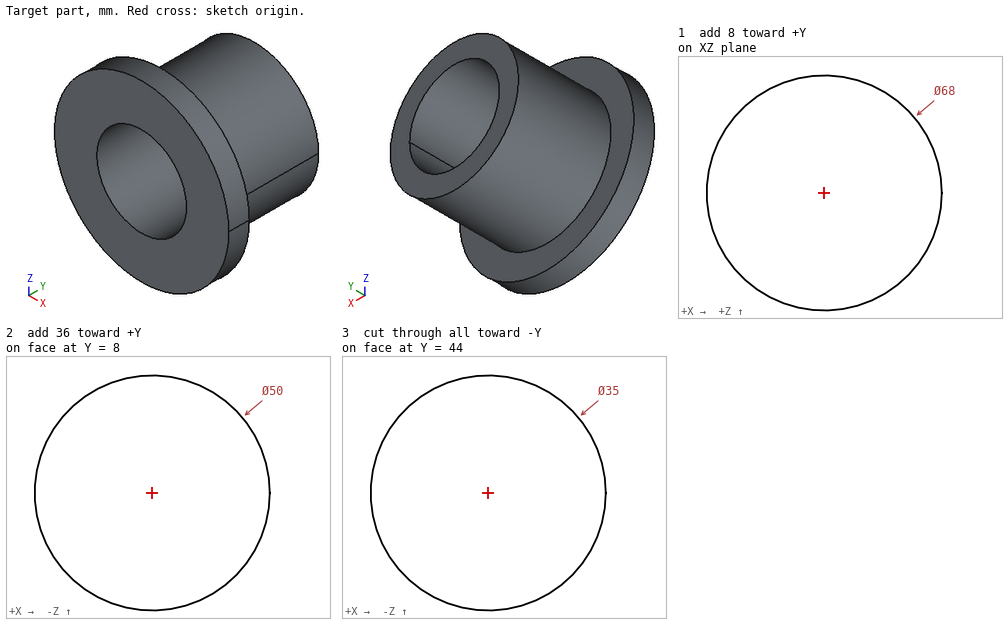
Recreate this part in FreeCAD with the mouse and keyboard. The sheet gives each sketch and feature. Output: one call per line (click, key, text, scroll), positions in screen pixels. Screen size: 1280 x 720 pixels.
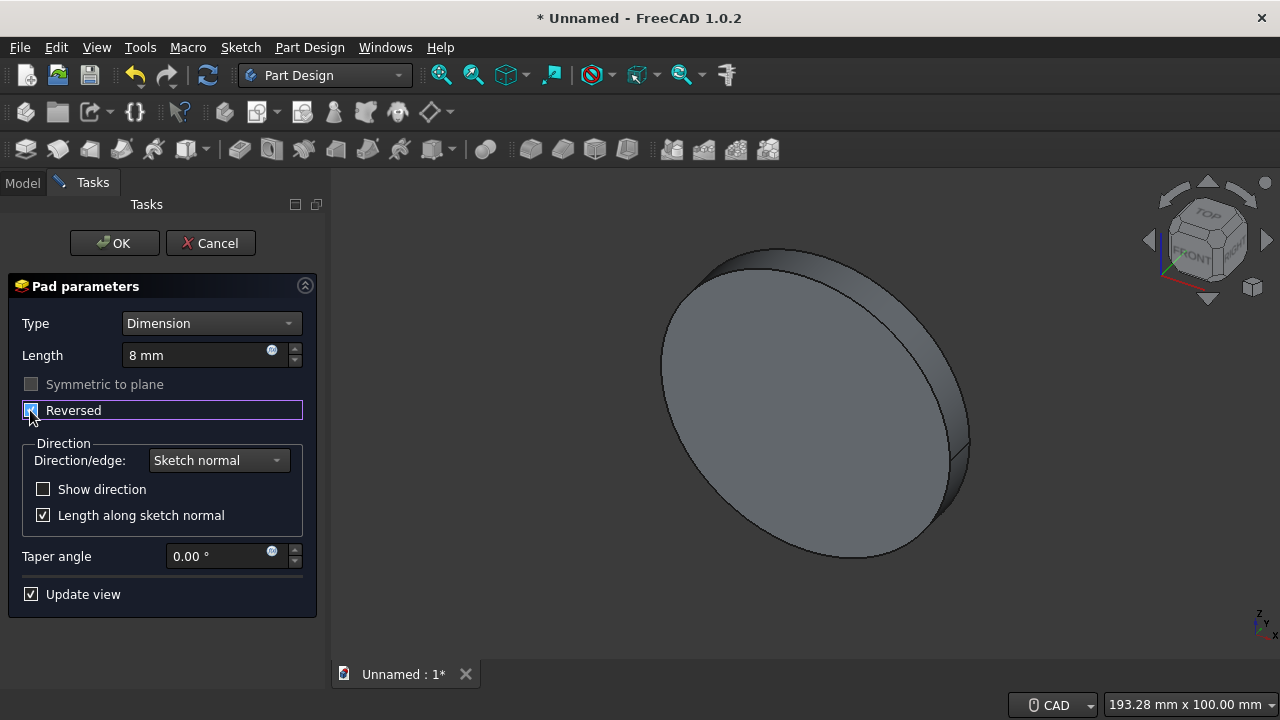
click(115, 243)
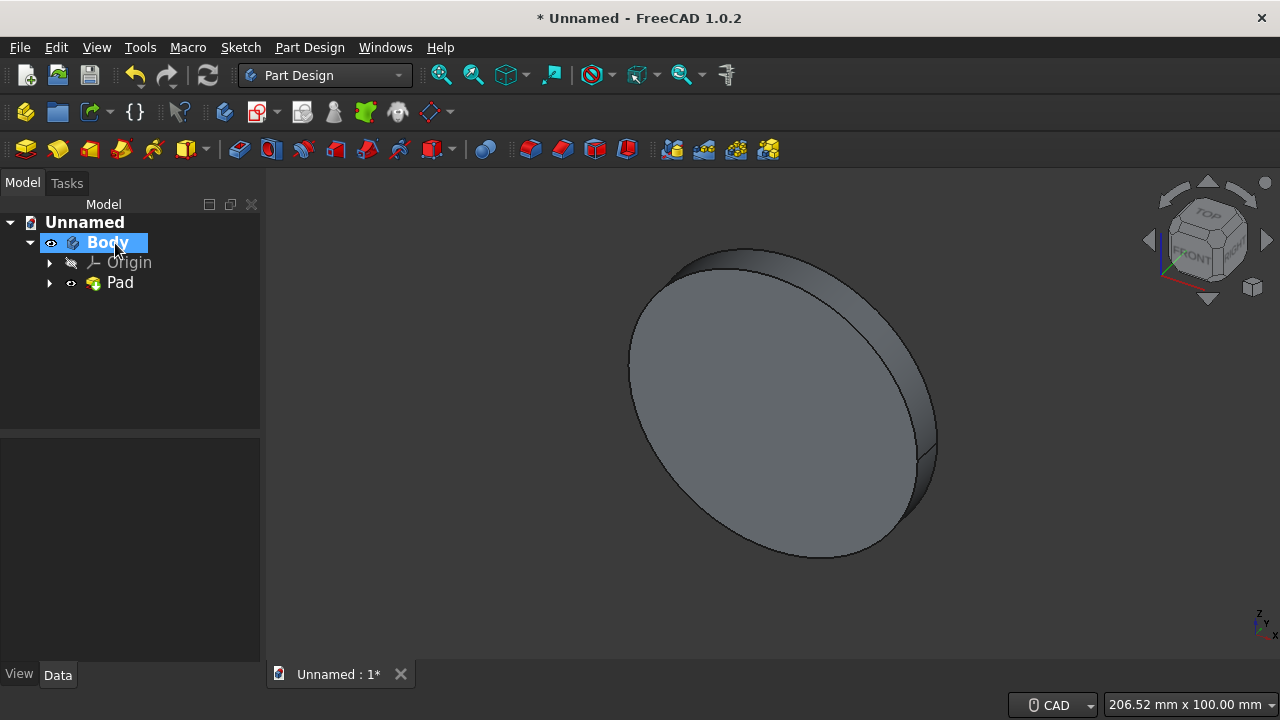
key(4)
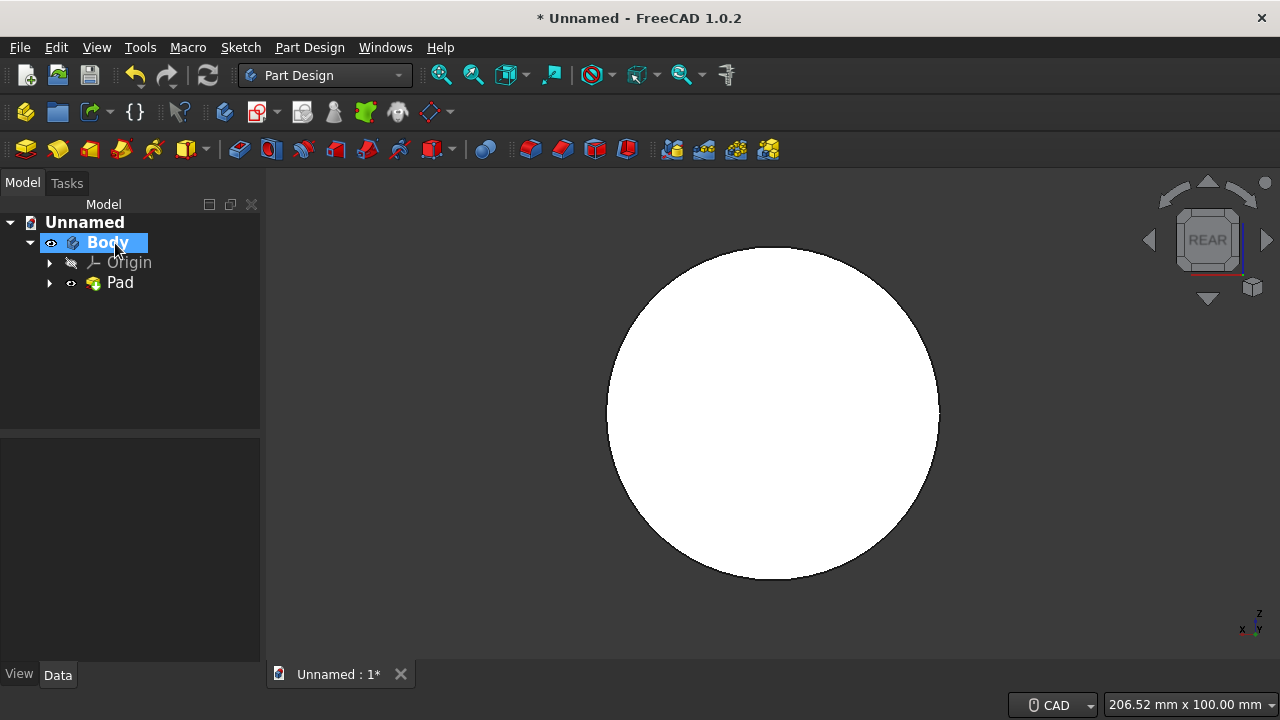
click(773, 412)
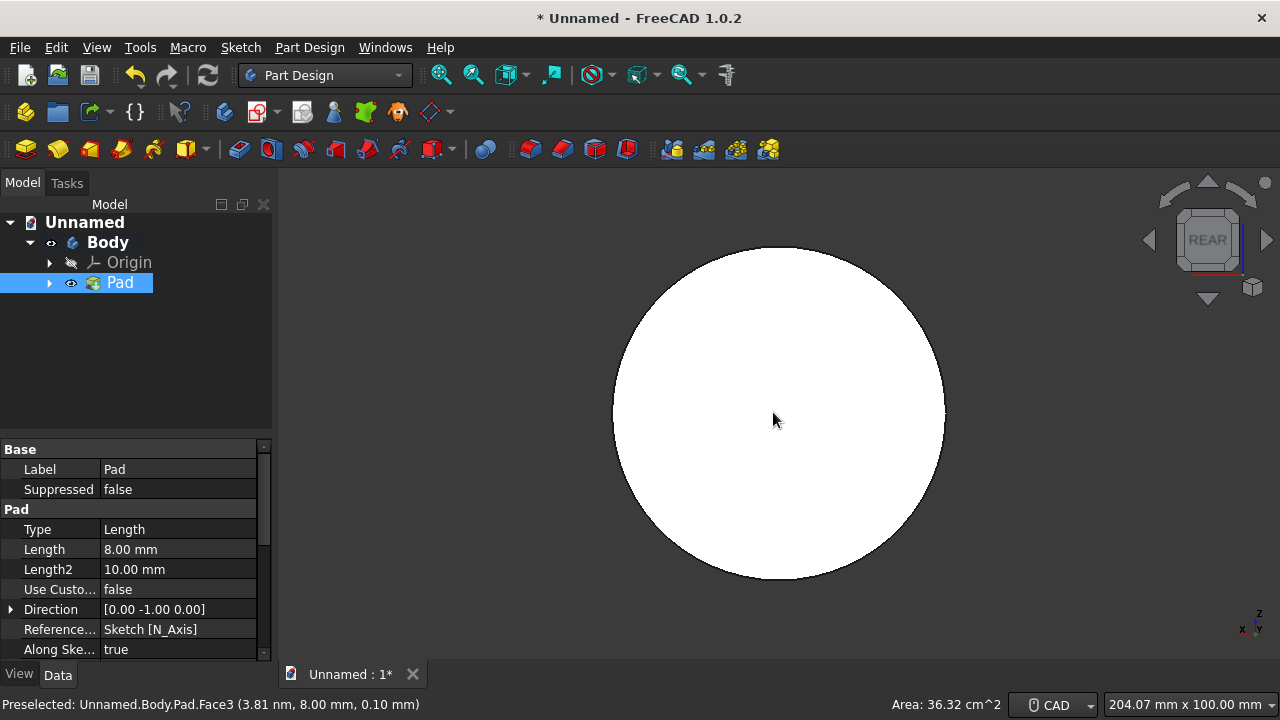
click(258, 112)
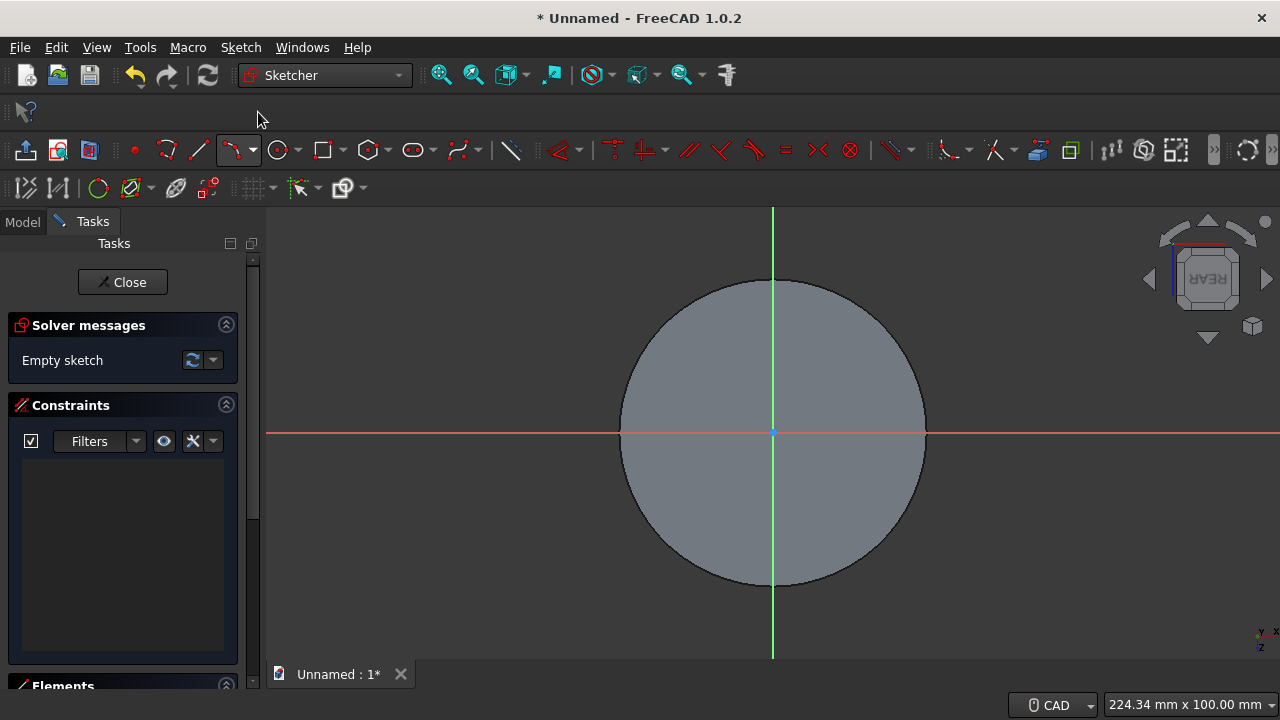
key(g)
key(c)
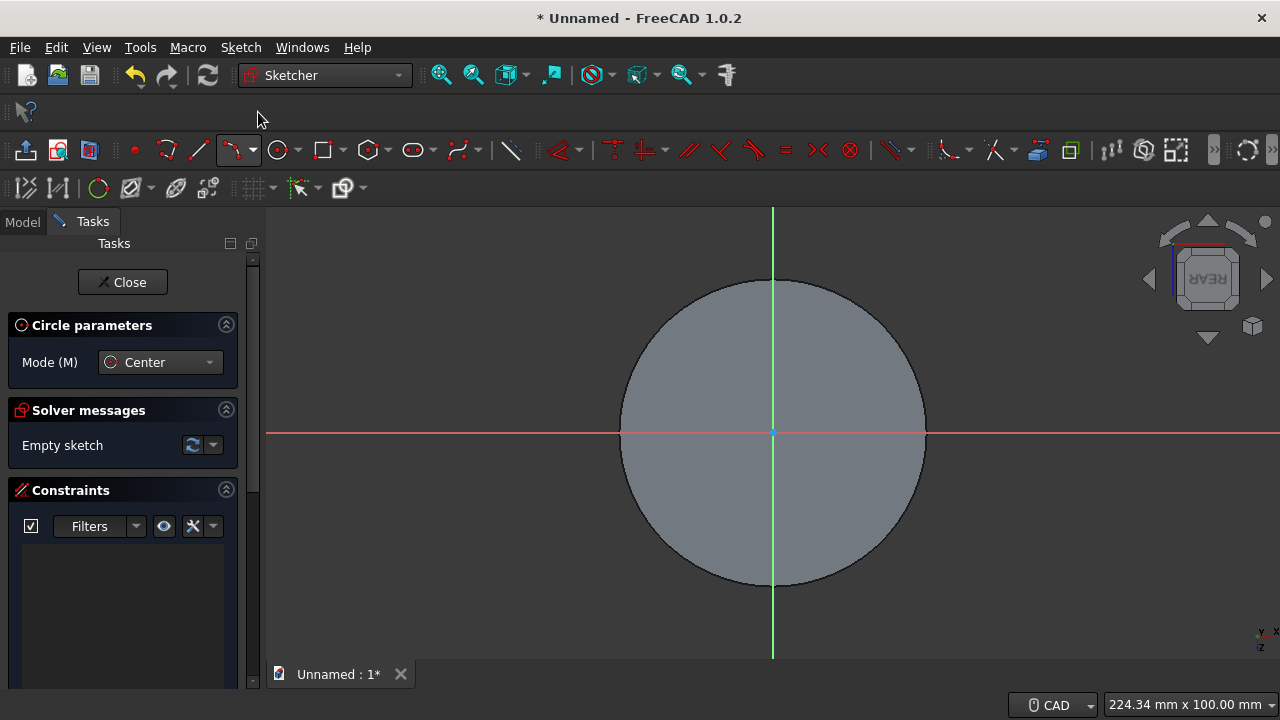
click(773, 433)
move(853, 353)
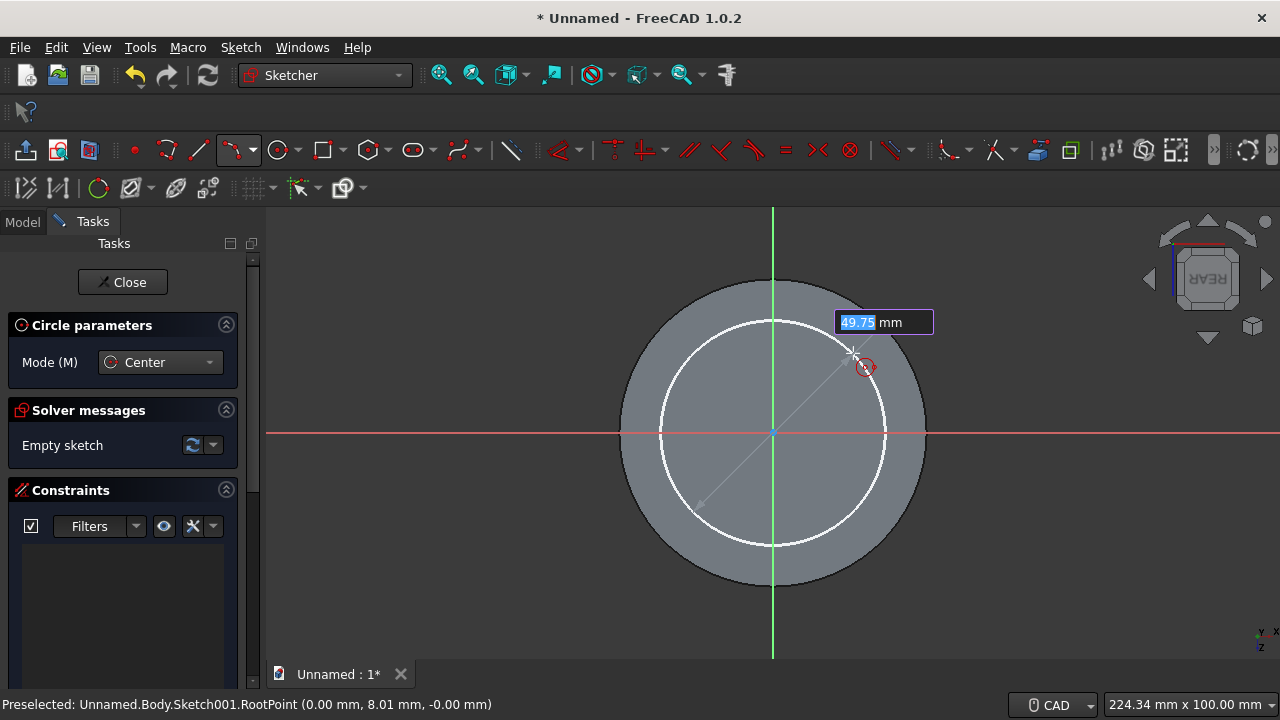
text(50)
key(Return)
key(Escape)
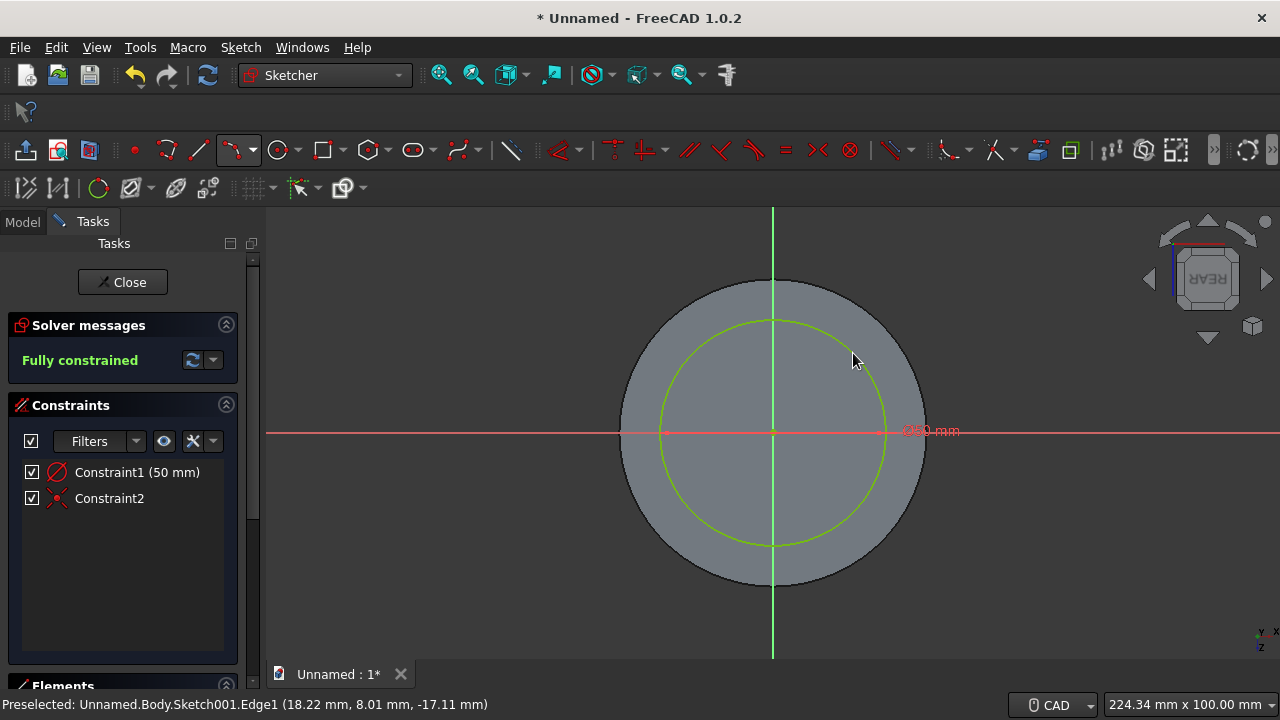
click(123, 282)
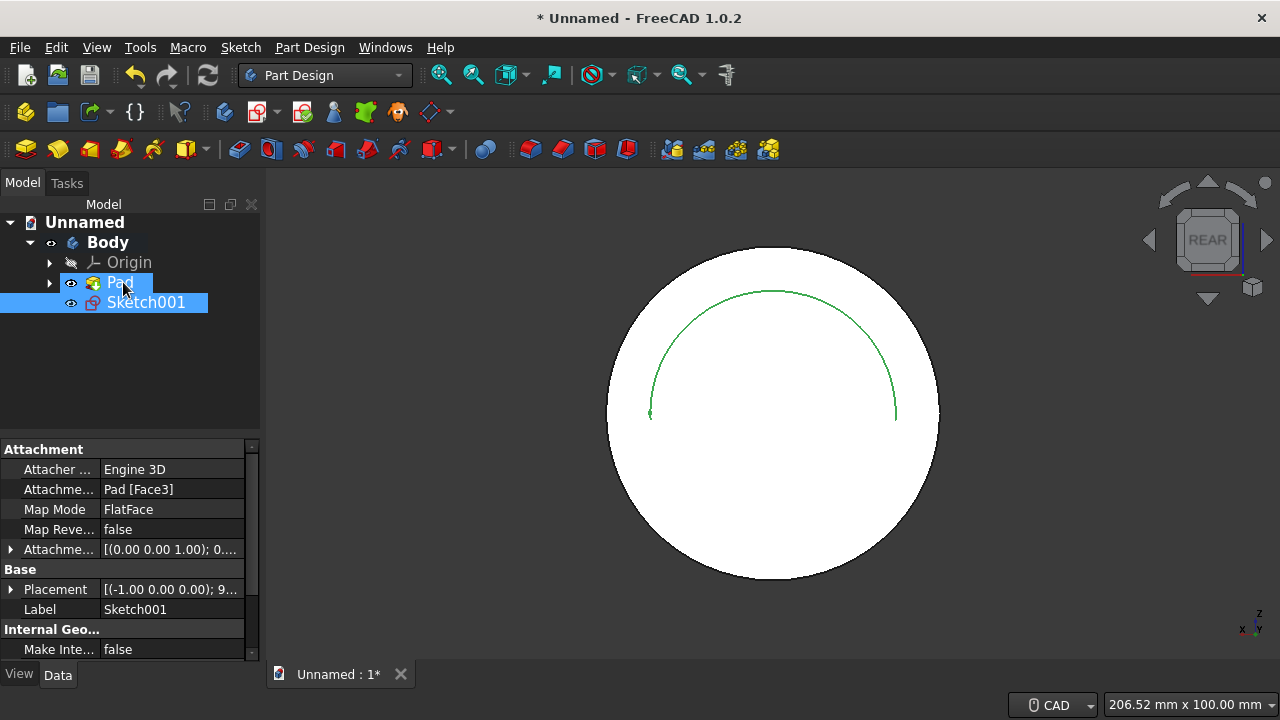
click(26, 150)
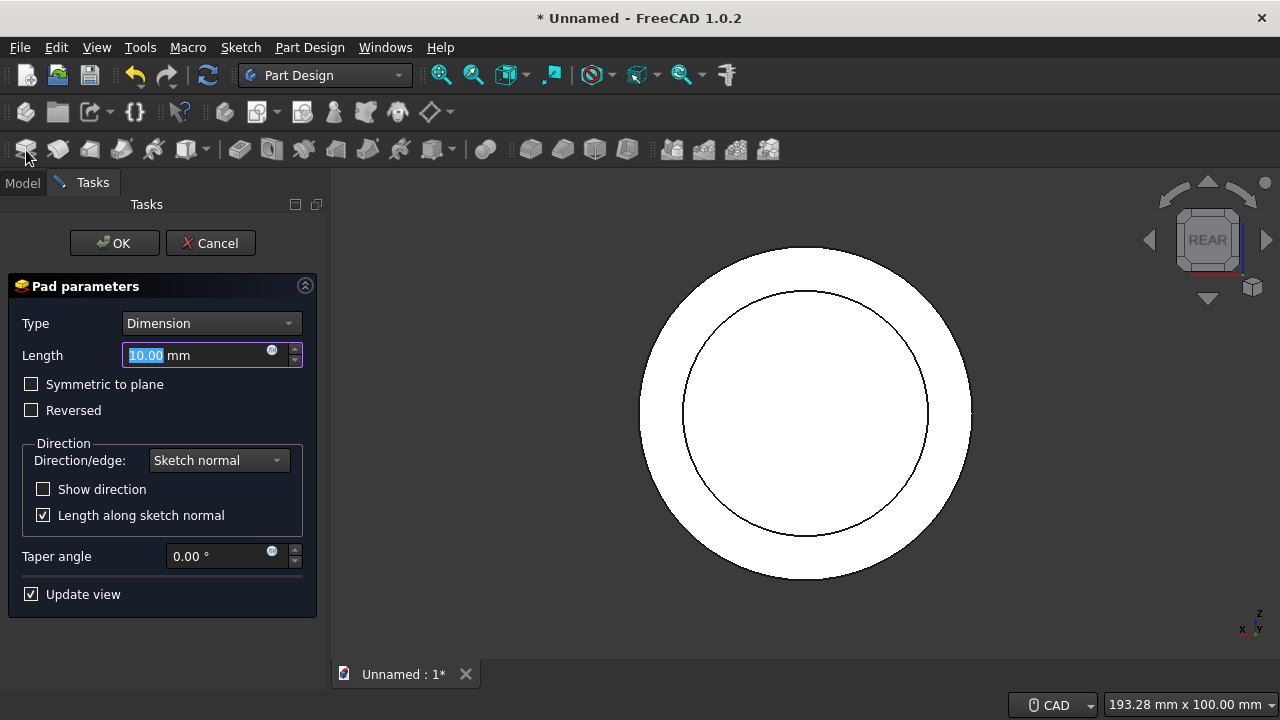
text(36)
key(Tab)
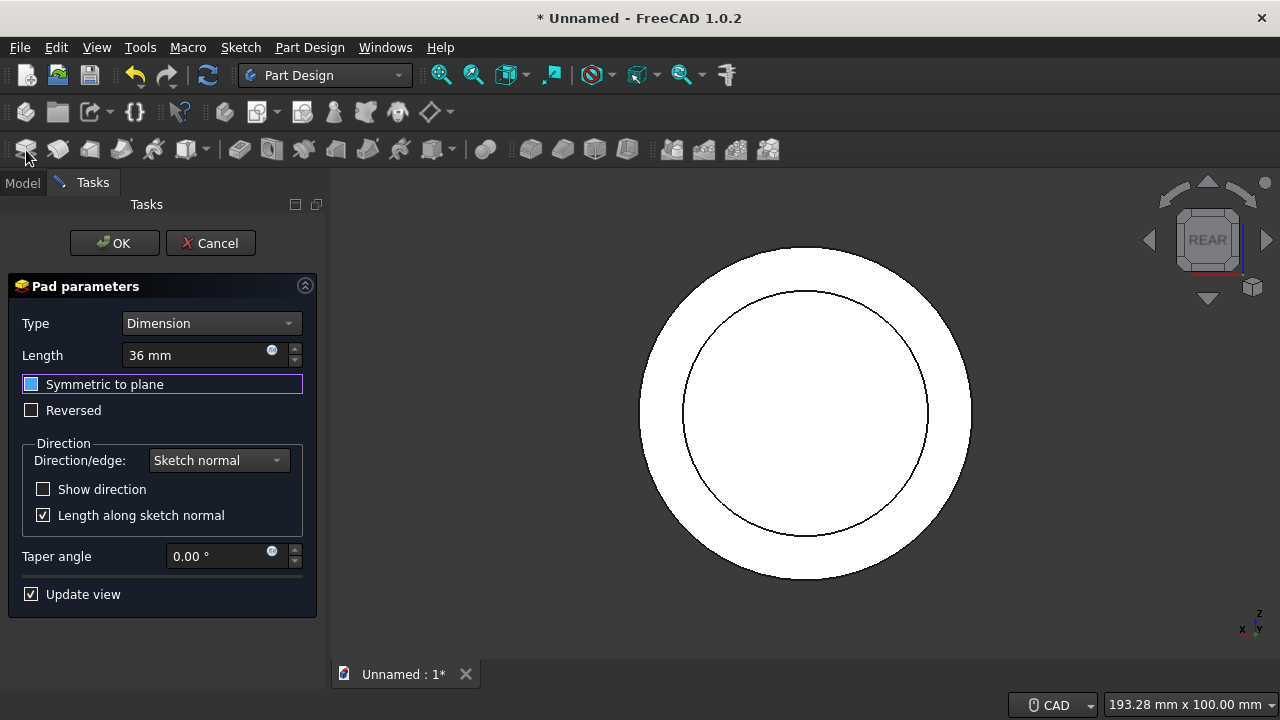
click(115, 243)